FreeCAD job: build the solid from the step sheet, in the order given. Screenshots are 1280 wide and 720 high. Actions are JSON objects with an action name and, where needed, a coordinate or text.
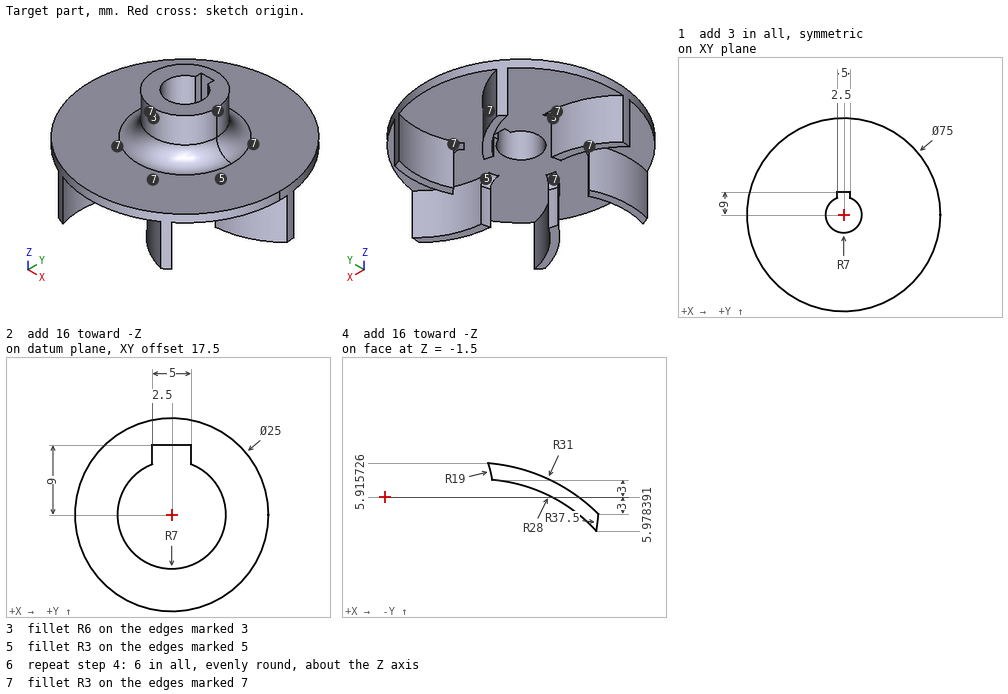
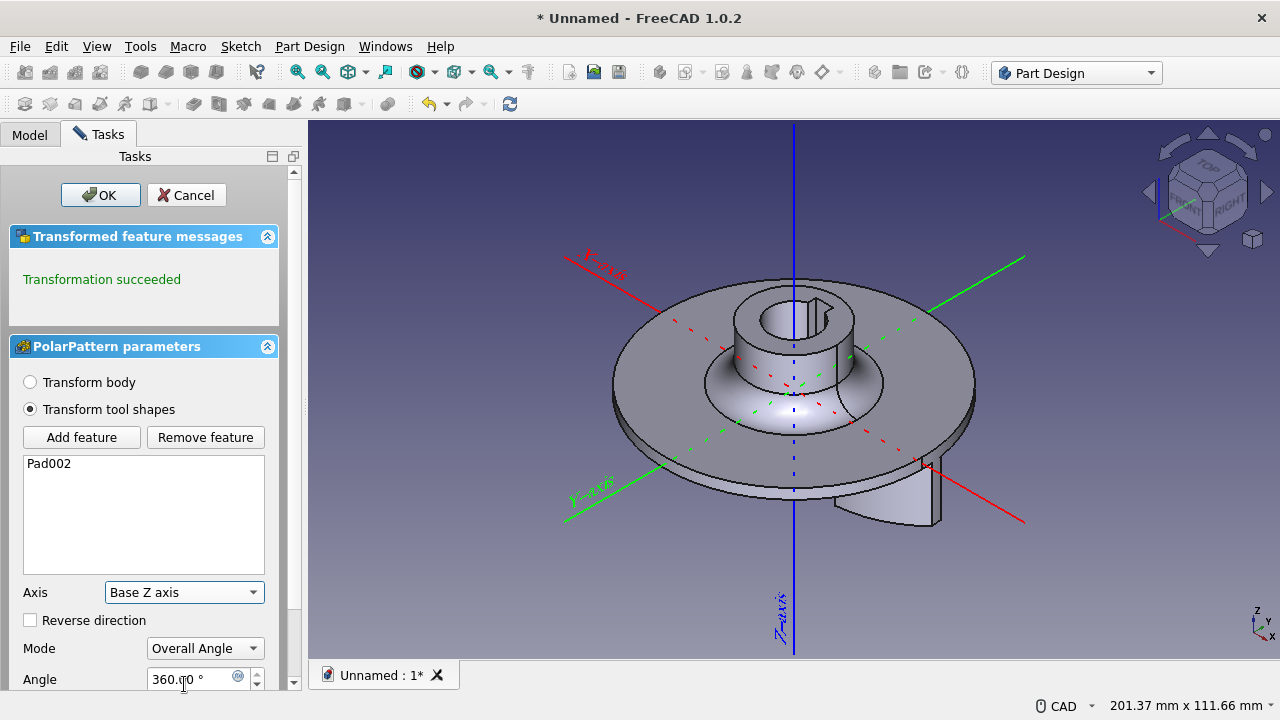
{"action": "scroll", "coordinate": [294, 428], "scroll_direction": "down", "scroll_amount": 2}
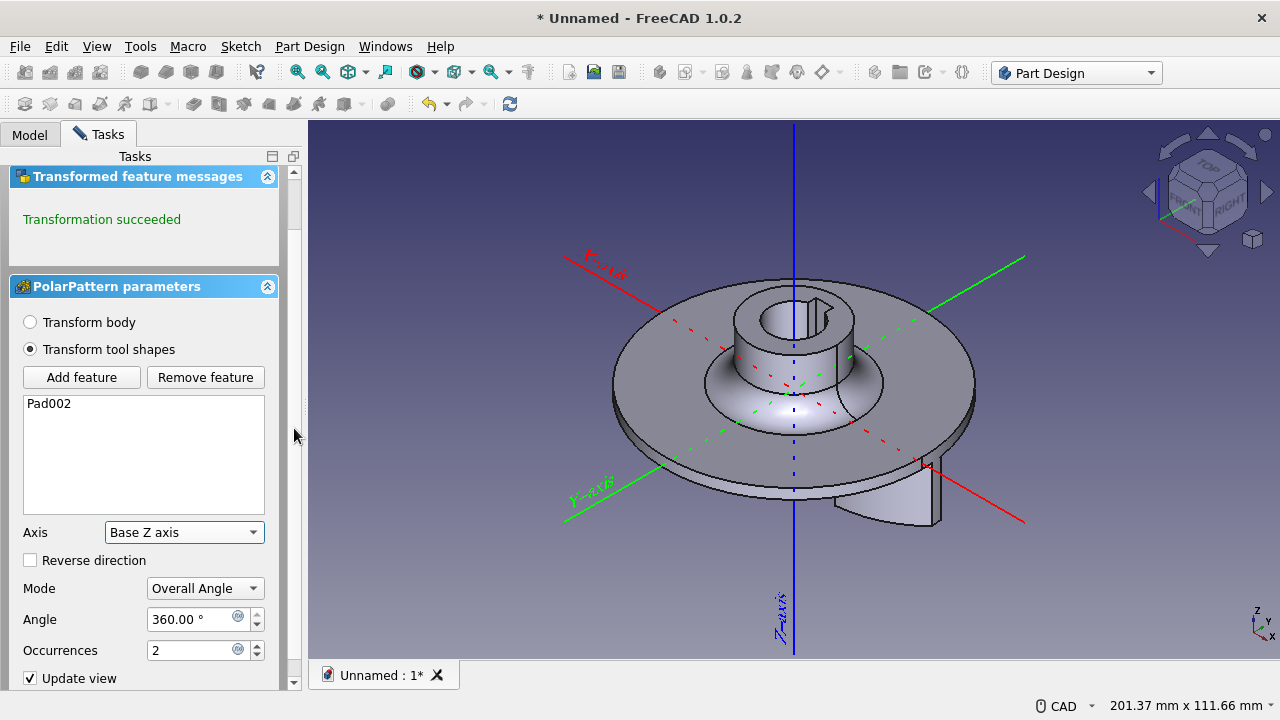
{"action": "triple_click", "coordinate": [199, 630]}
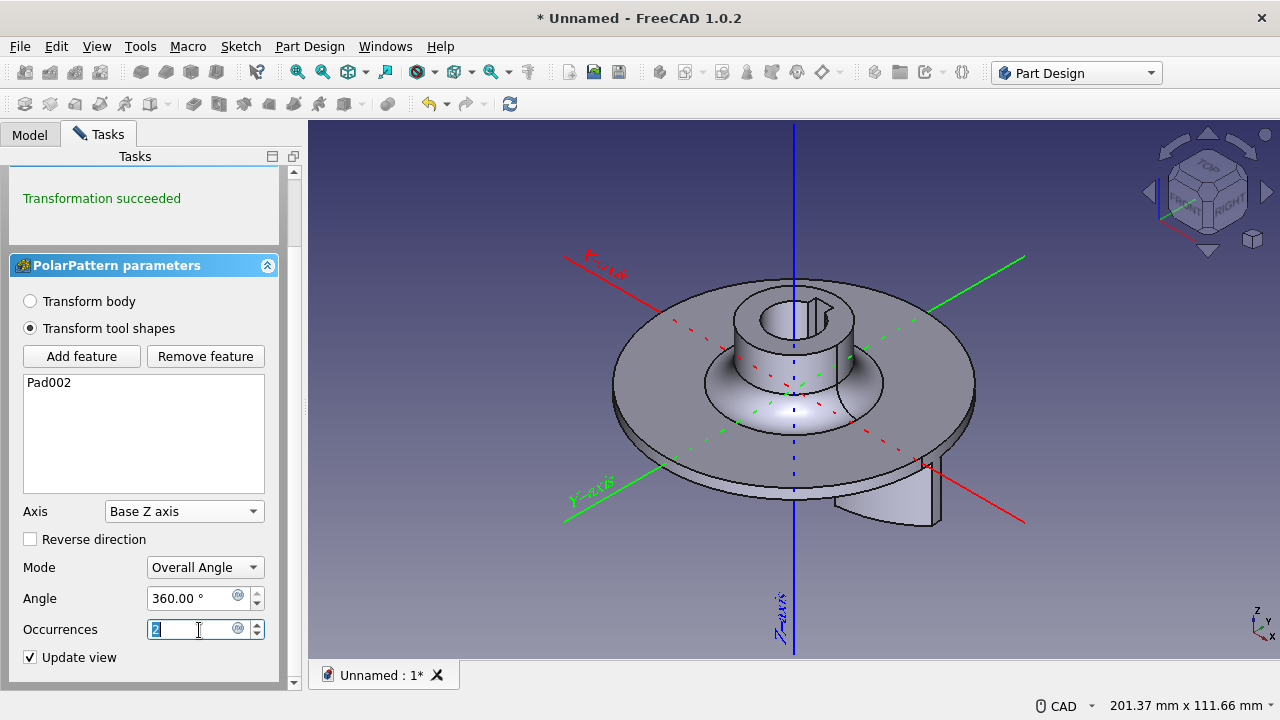
{"action": "type", "text": "6"}
{"action": "key", "text": "Tab"}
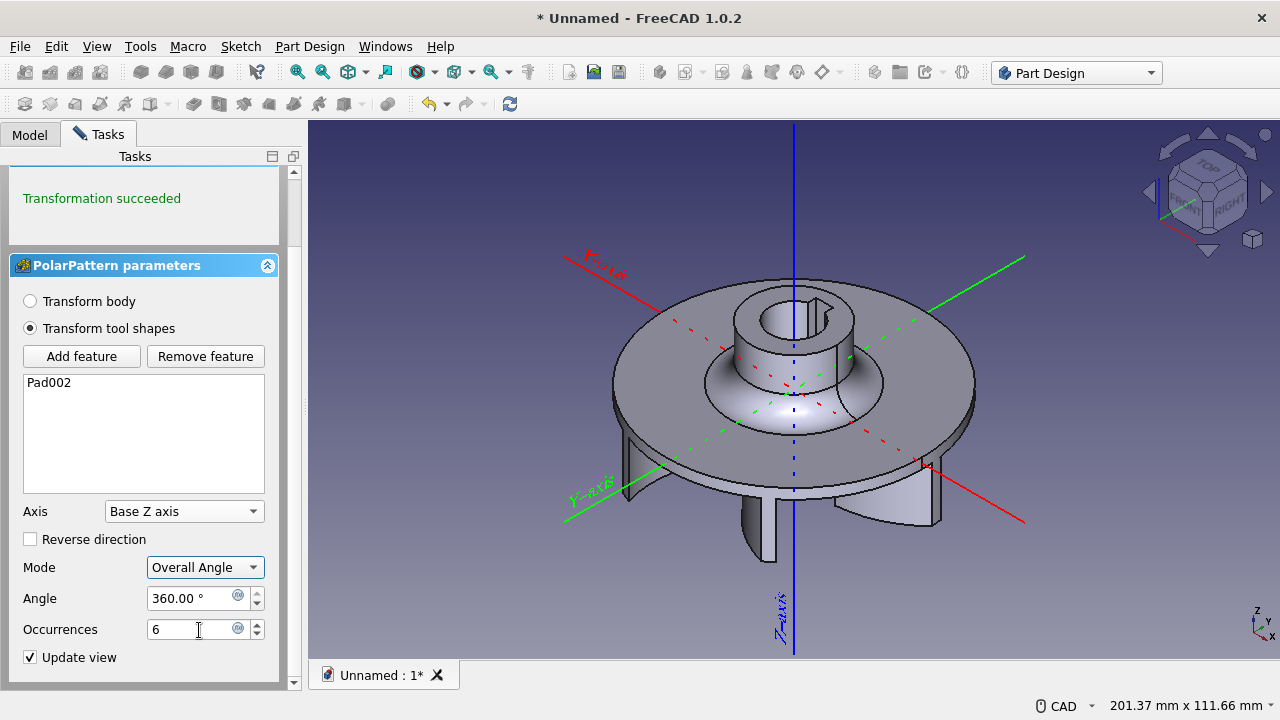
{"action": "scroll", "coordinate": [294, 428], "scroll_direction": "up", "scroll_amount": 3}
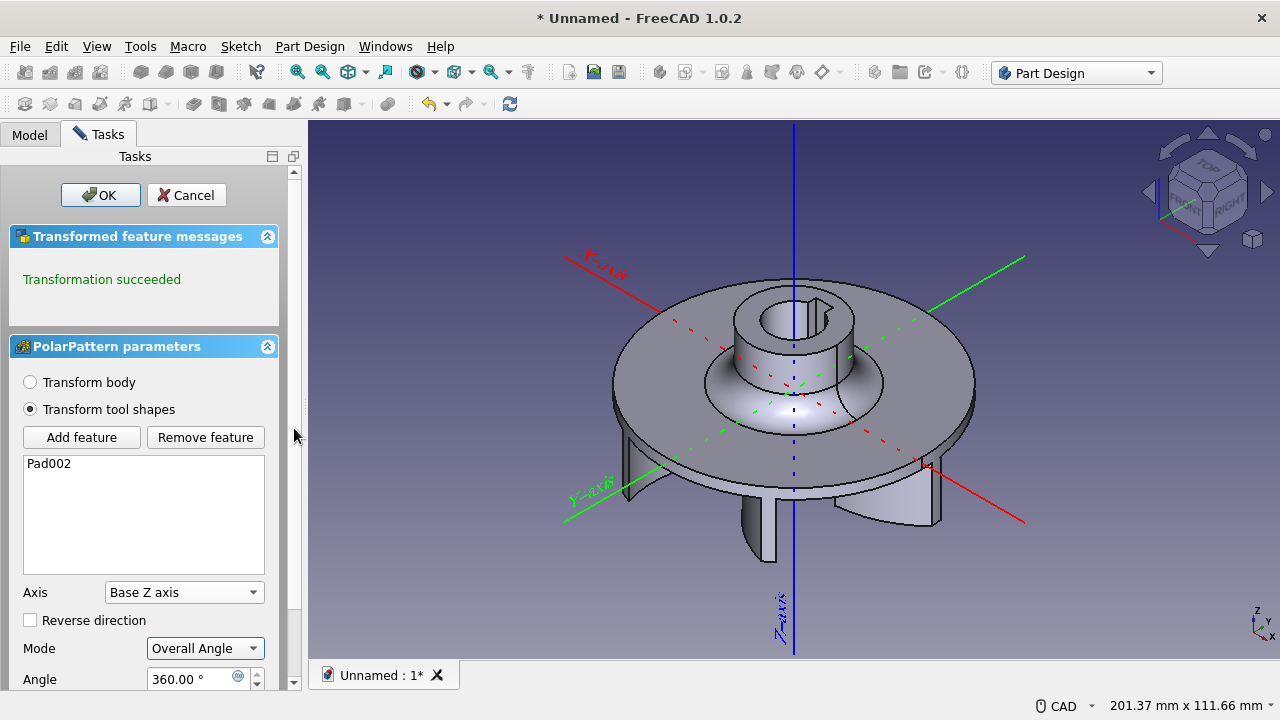
{"action": "left_click", "coordinate": [101, 195]}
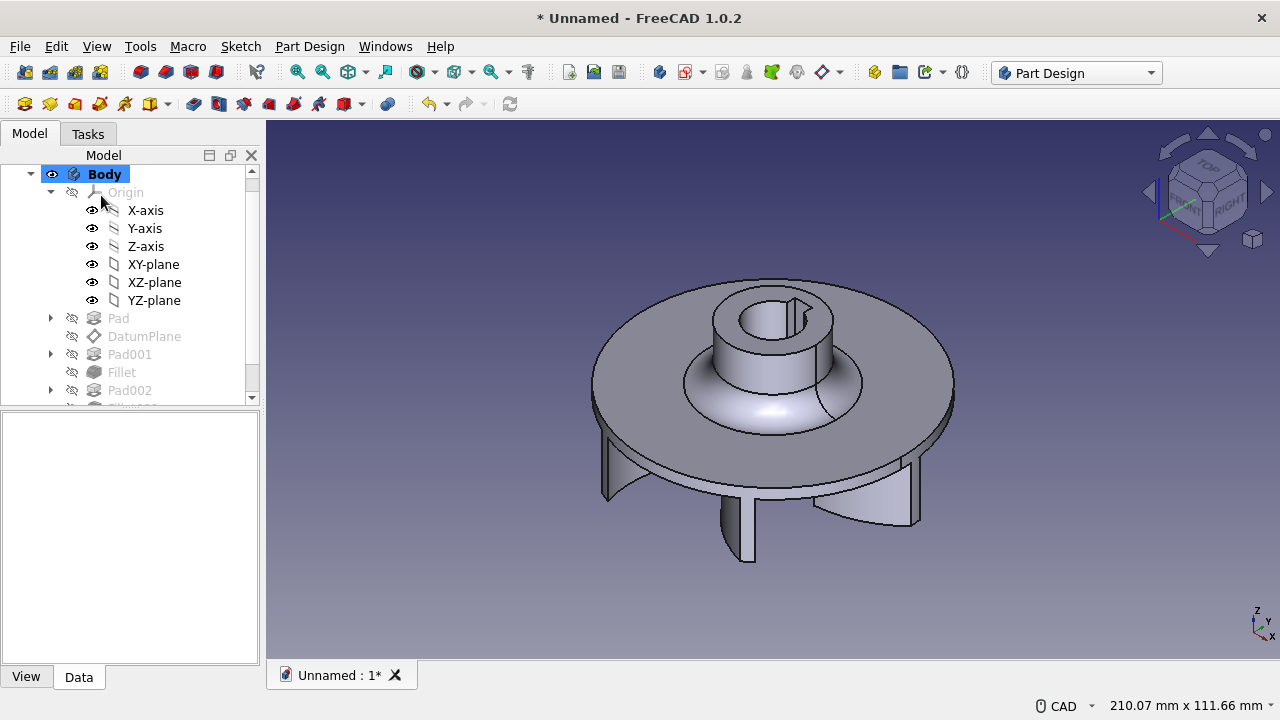
{"action": "scroll", "coordinate": [865, 393], "scroll_direction": "up", "scroll_amount": 6}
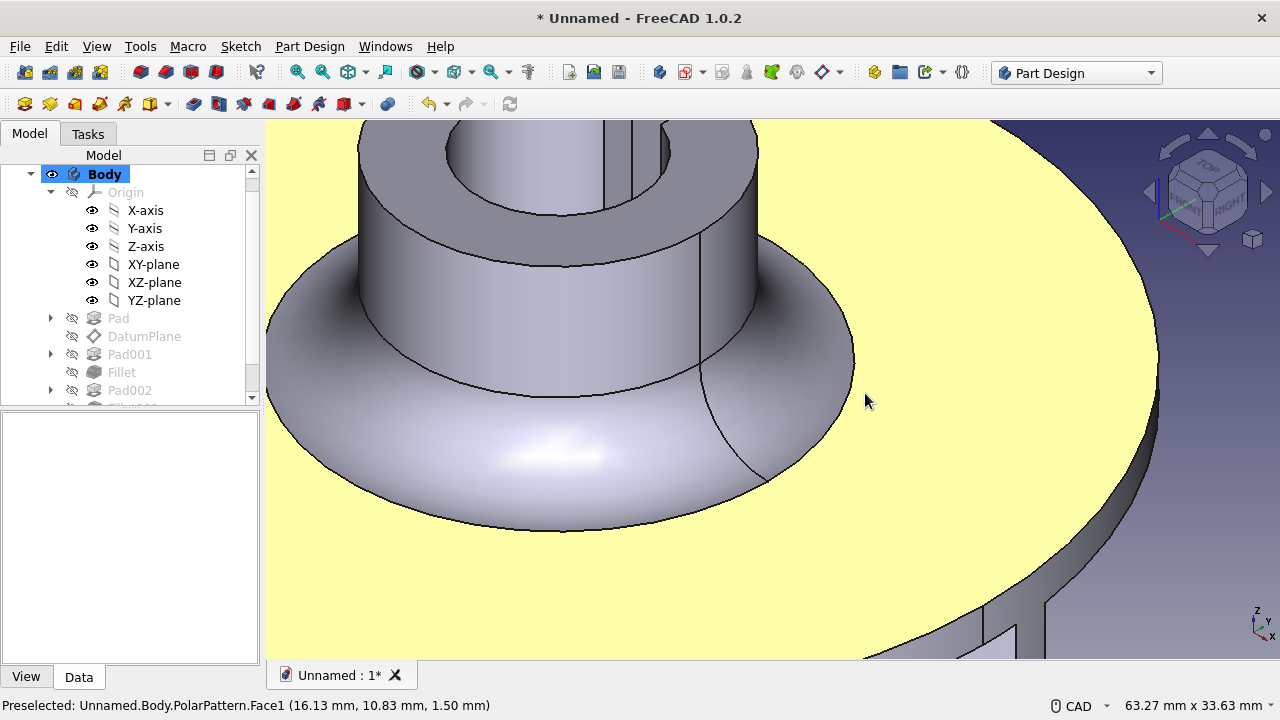
{"action": "left_click", "coordinate": [298, 72]}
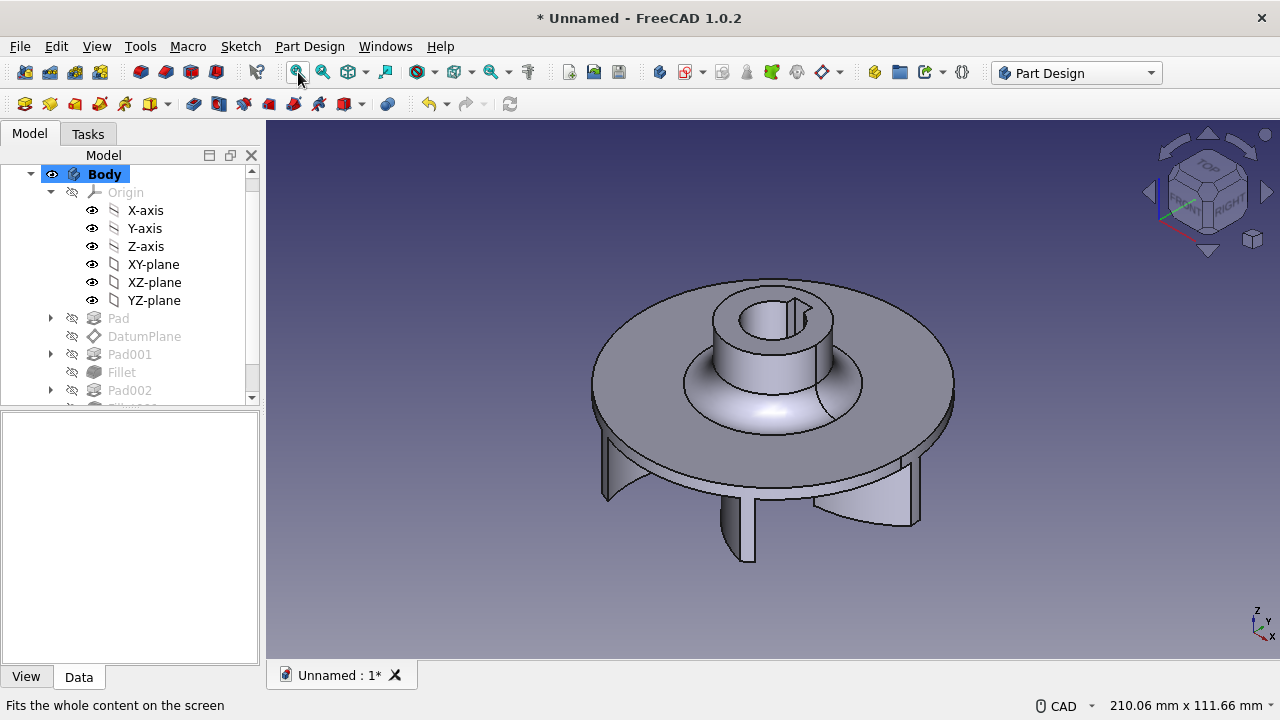
{"action": "key", "text": "2"}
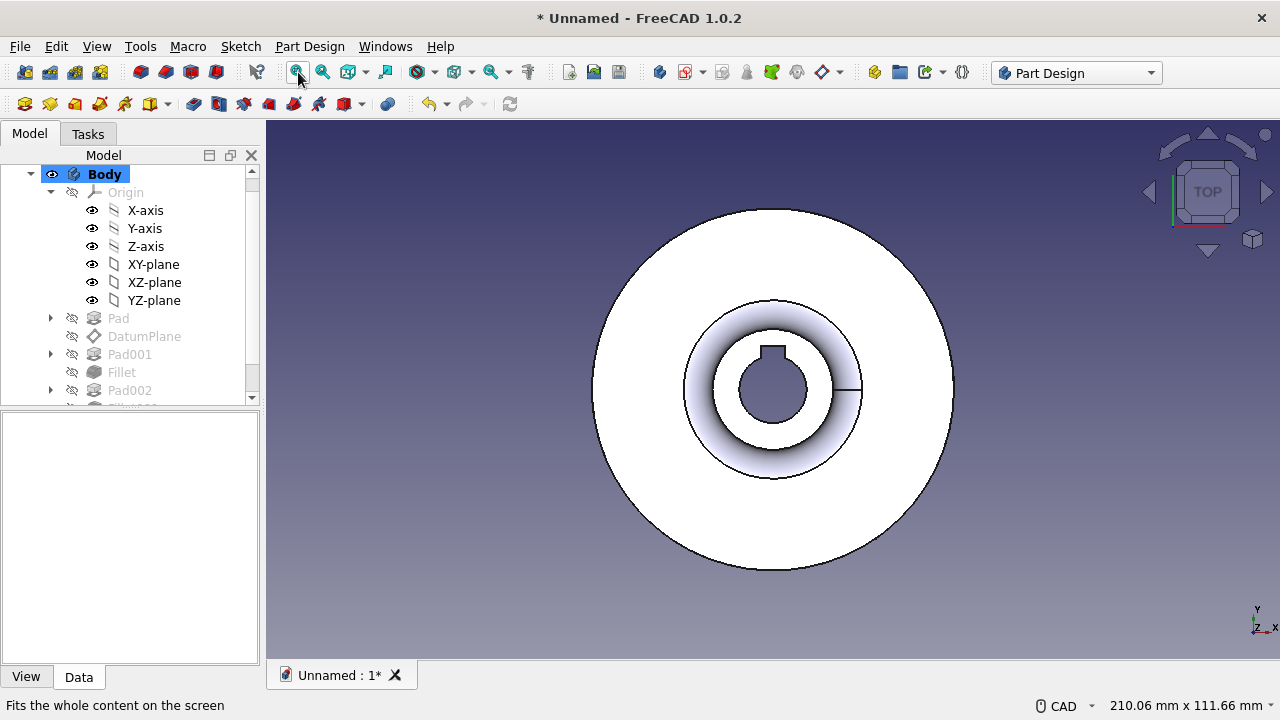
{"action": "scroll", "coordinate": [836, 322], "scroll_direction": "up", "scroll_amount": 6}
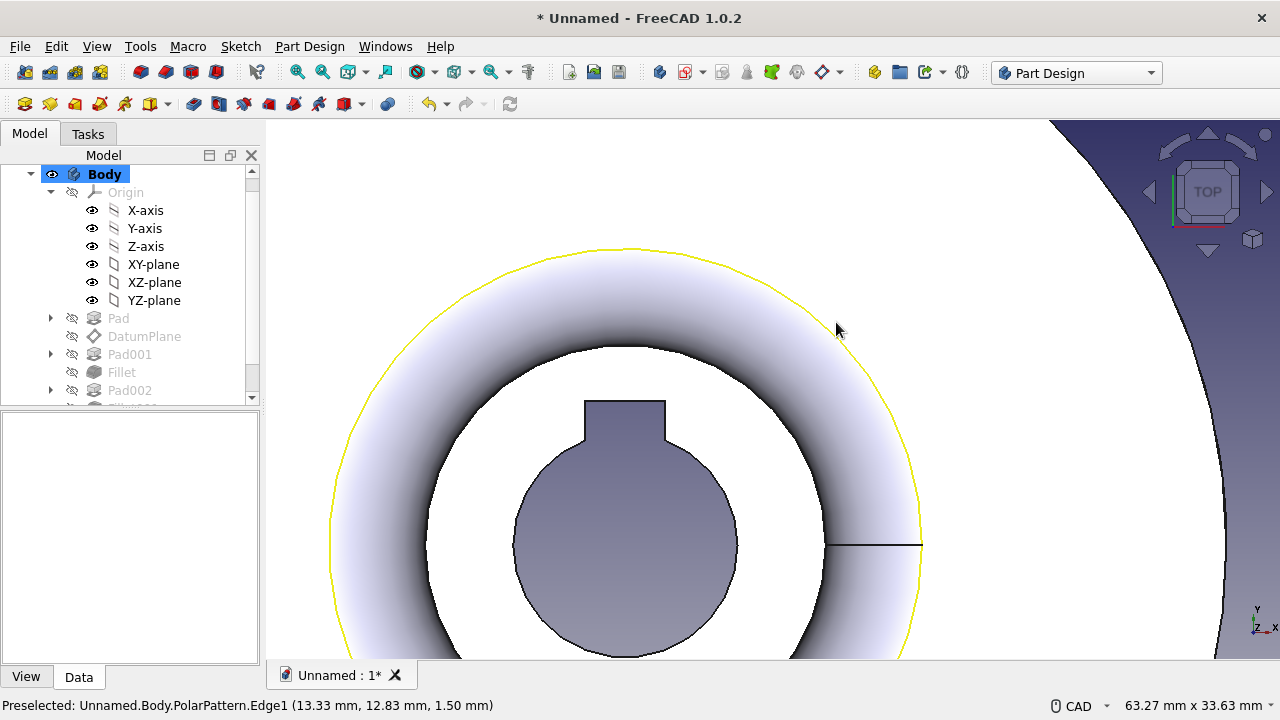
{"action": "left_click", "coordinate": [298, 72]}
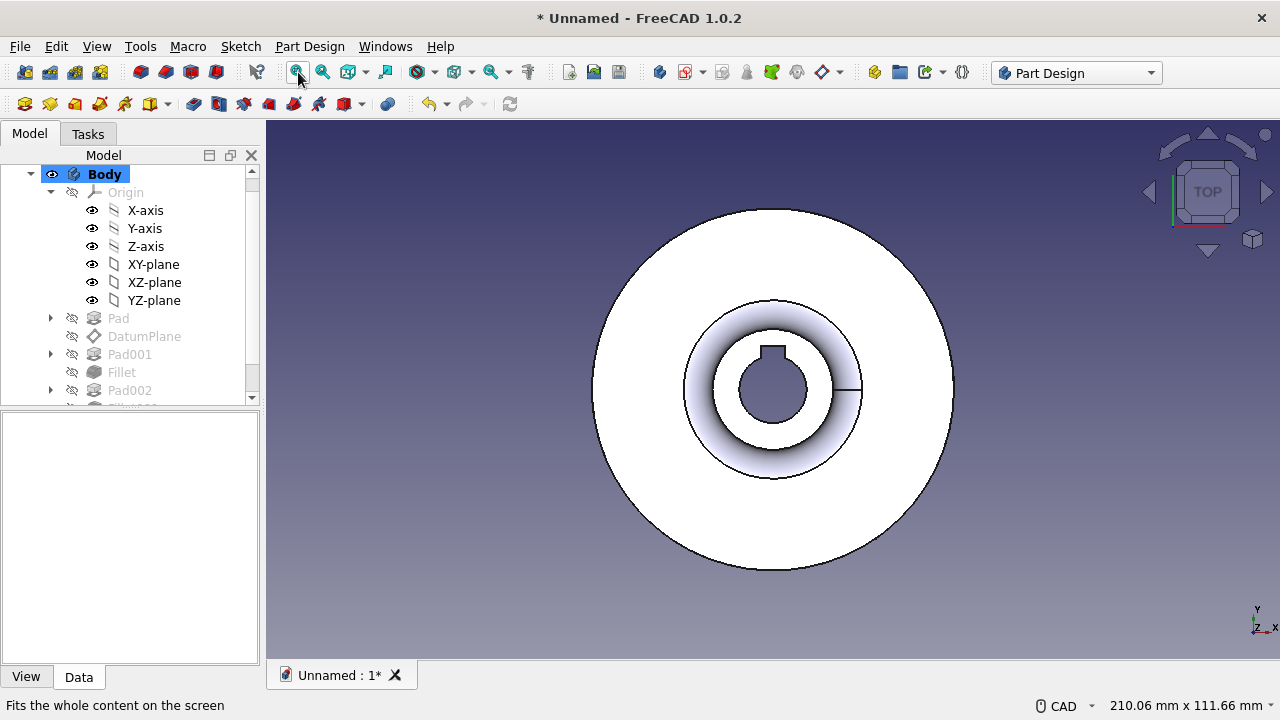
{"action": "key", "text": "0"}